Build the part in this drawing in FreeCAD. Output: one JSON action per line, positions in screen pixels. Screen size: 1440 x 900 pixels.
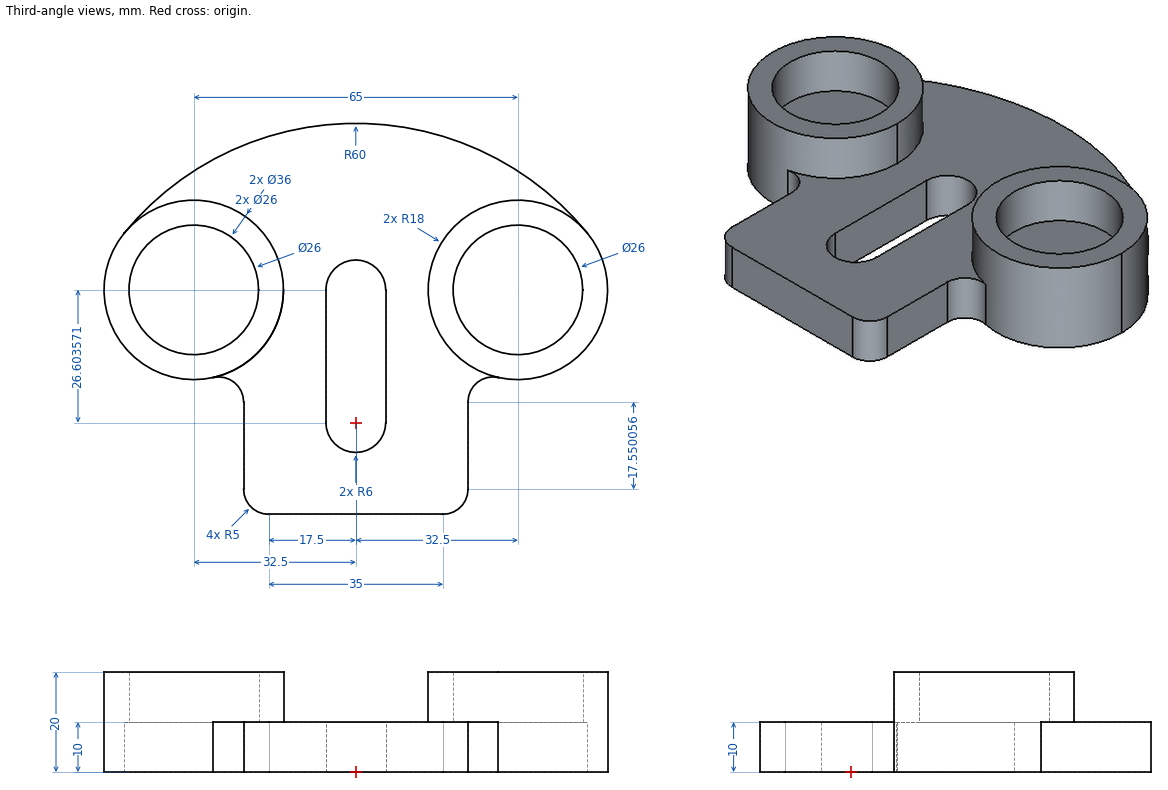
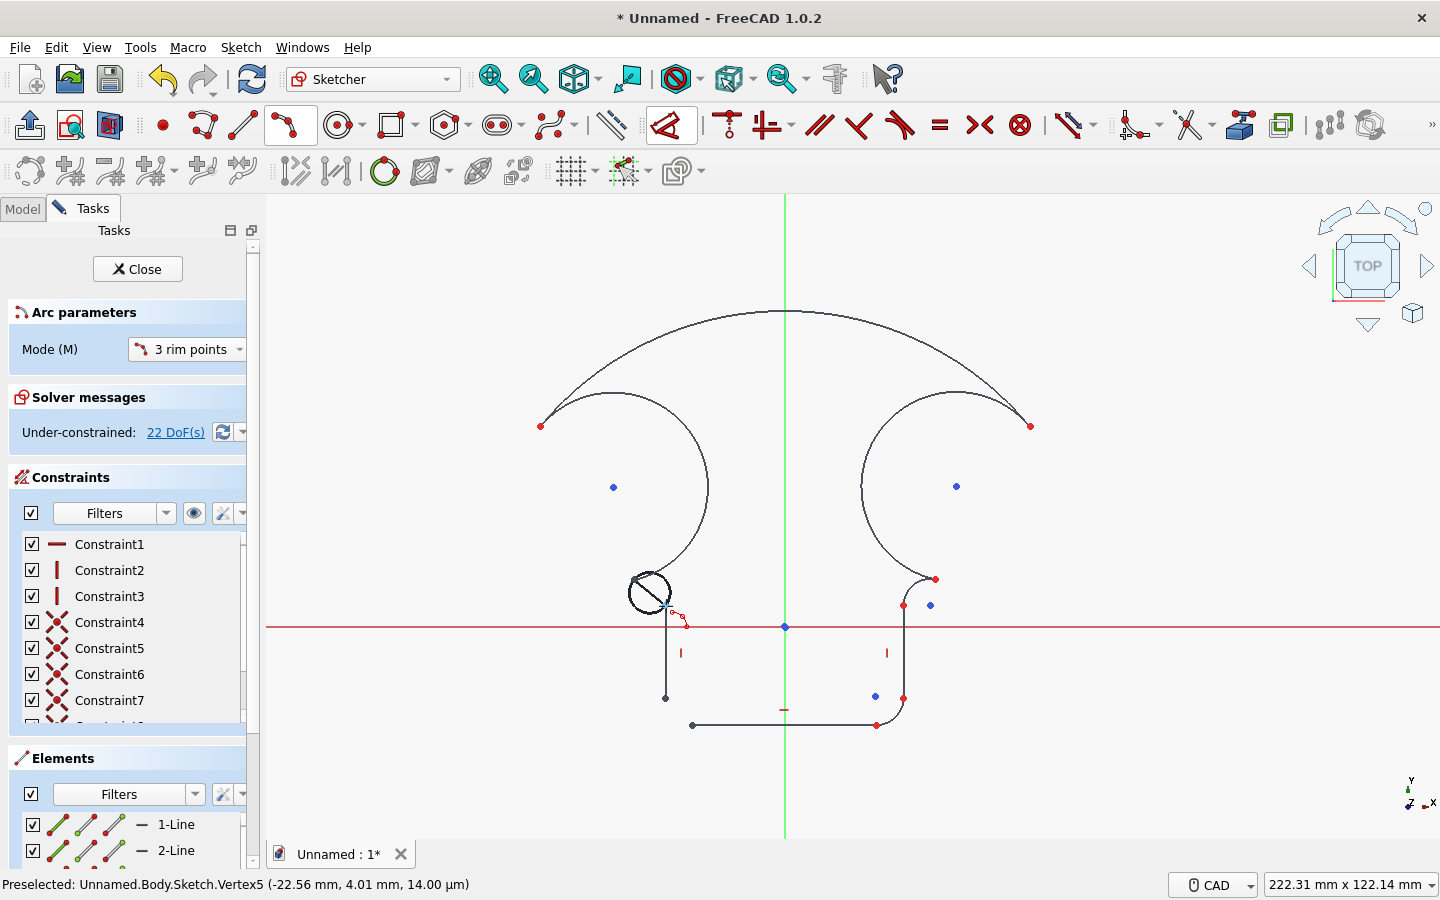
{"action": "scroll", "coordinate": [656, 584], "scroll_direction": "up", "scroll_amount": 3}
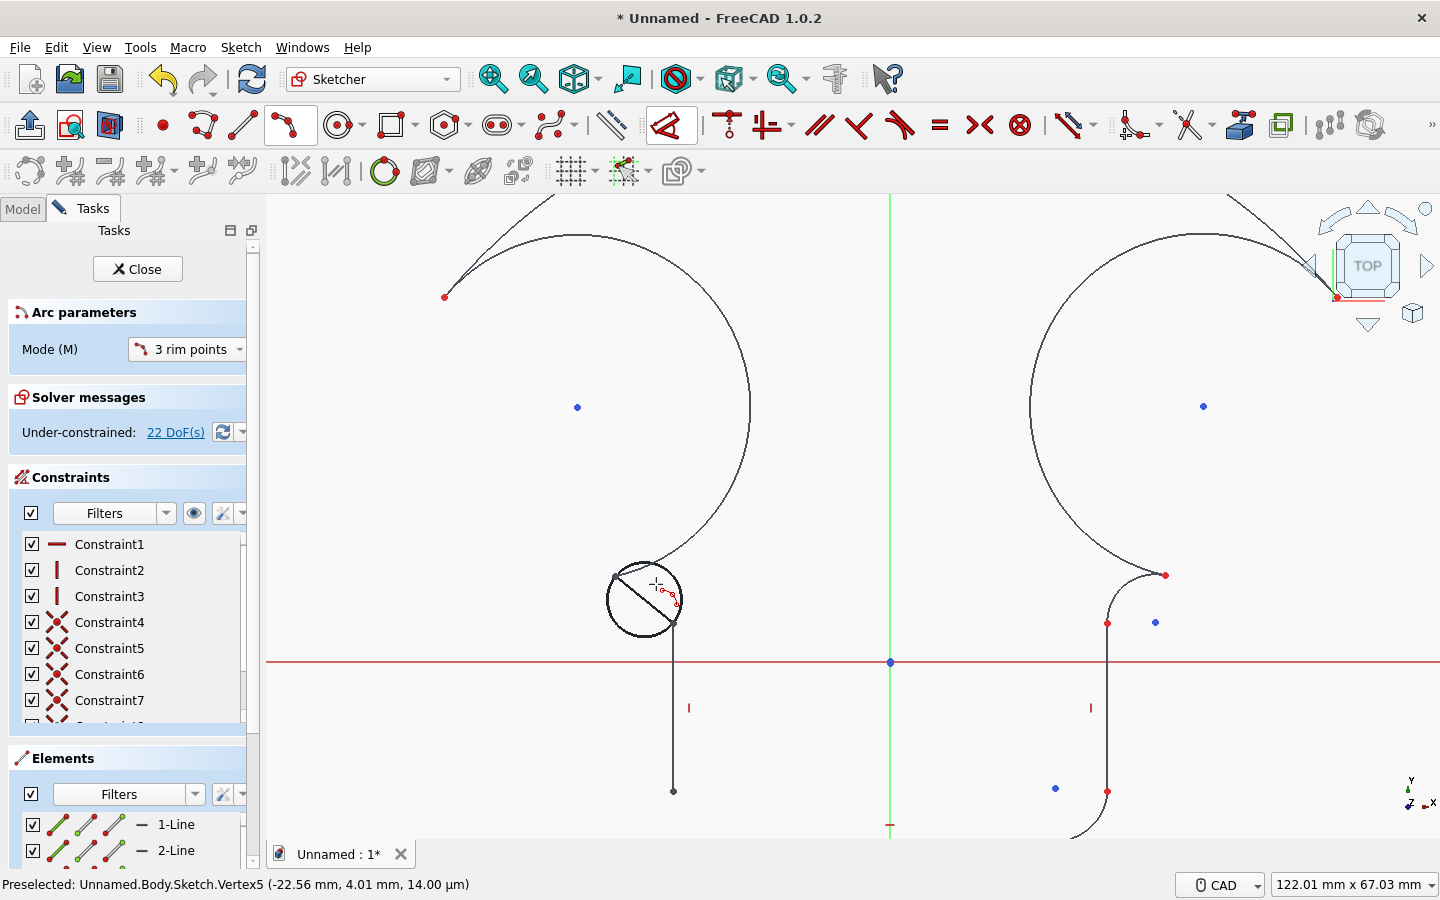
{"action": "left_click", "coordinate": [656, 584]}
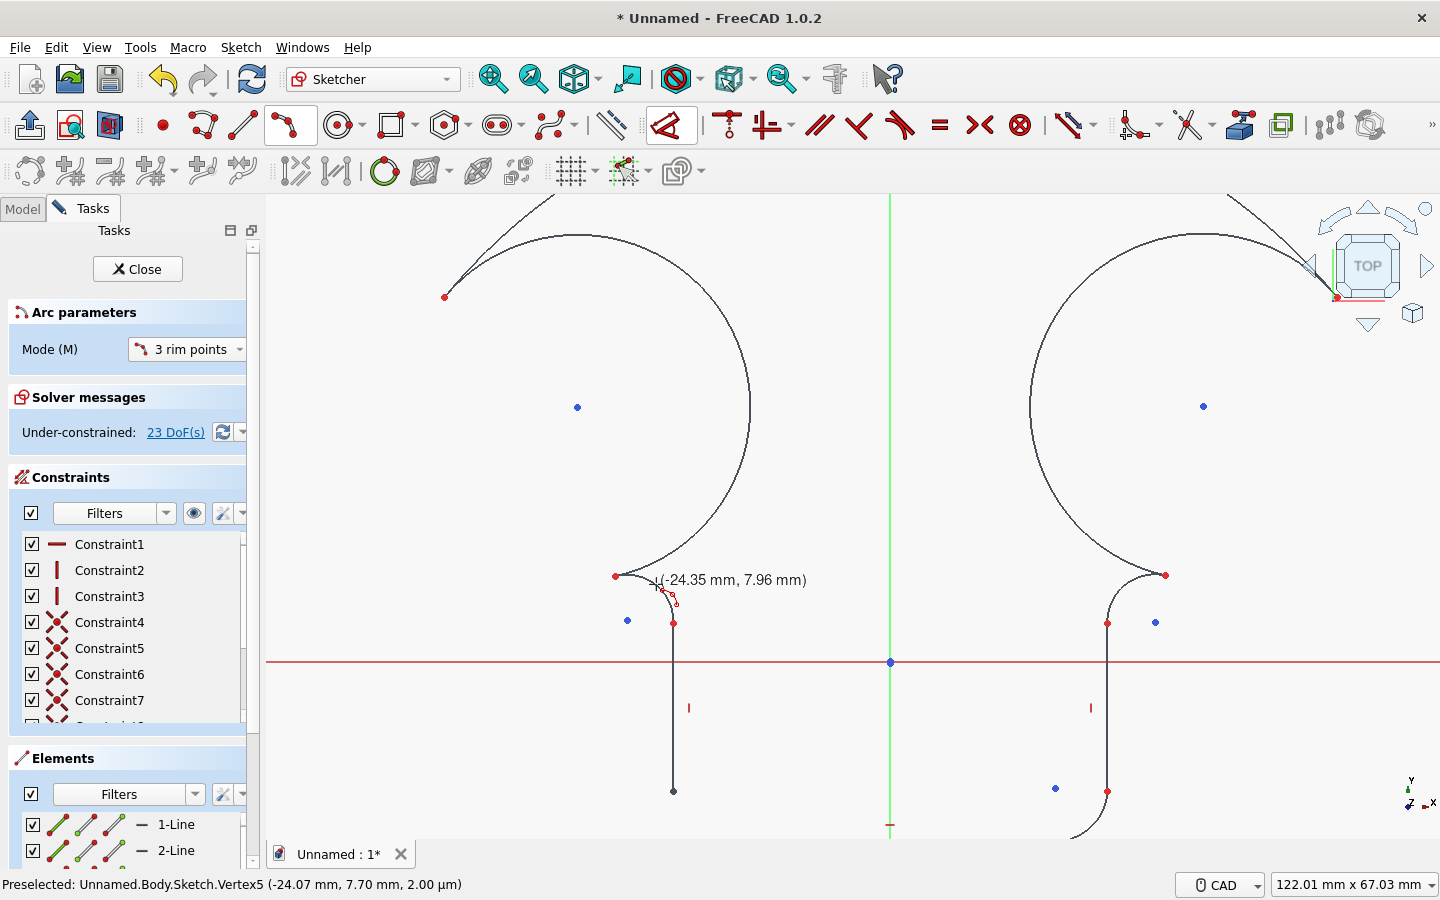
{"action": "left_click", "coordinate": [673, 792]}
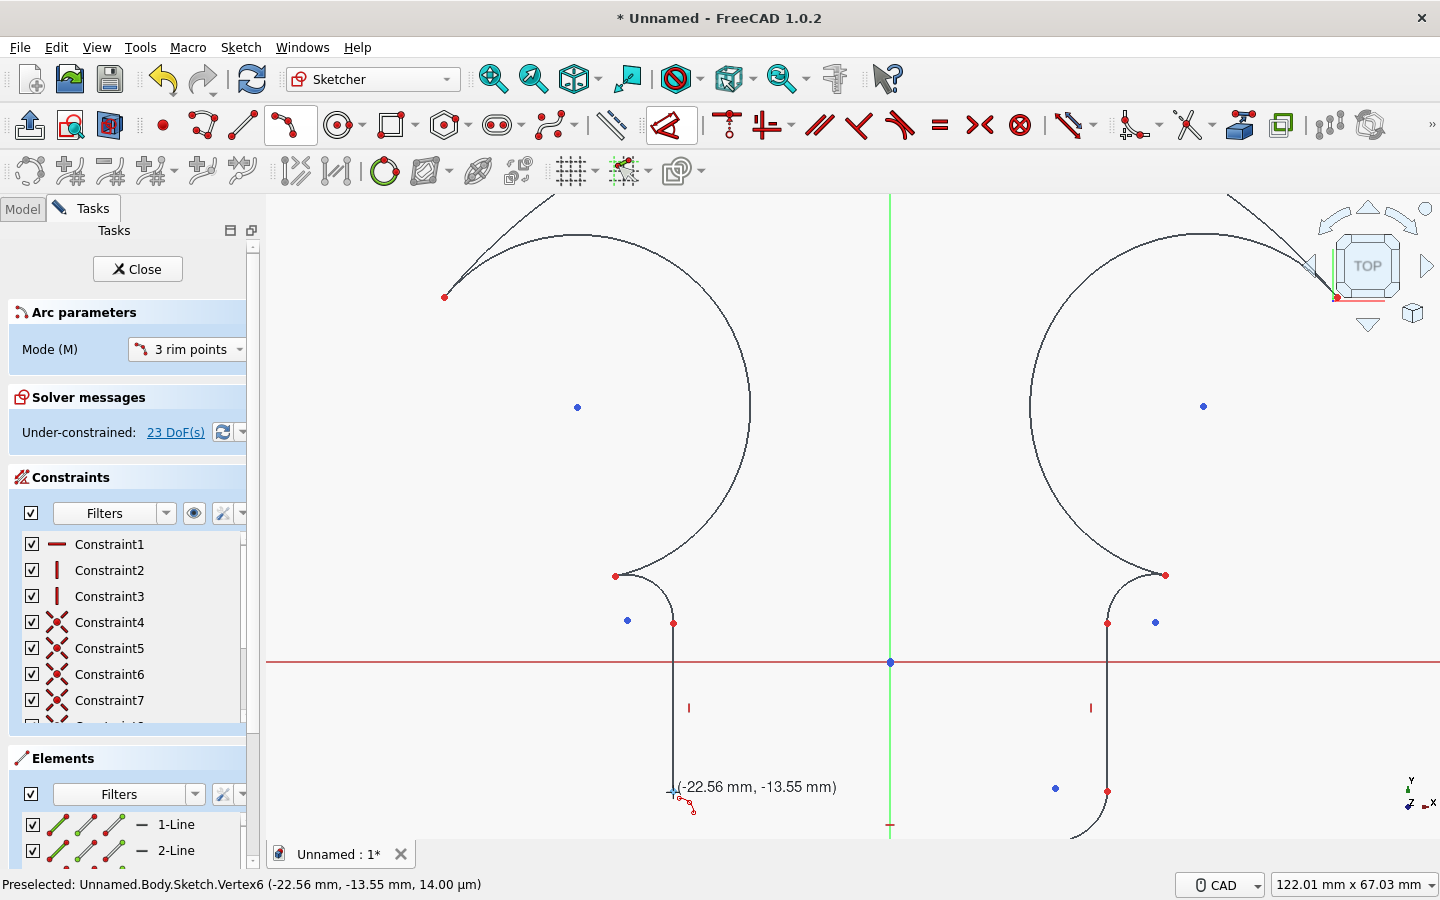
{"action": "scroll", "coordinate": [656, 583], "scroll_direction": "down", "scroll_amount": 3}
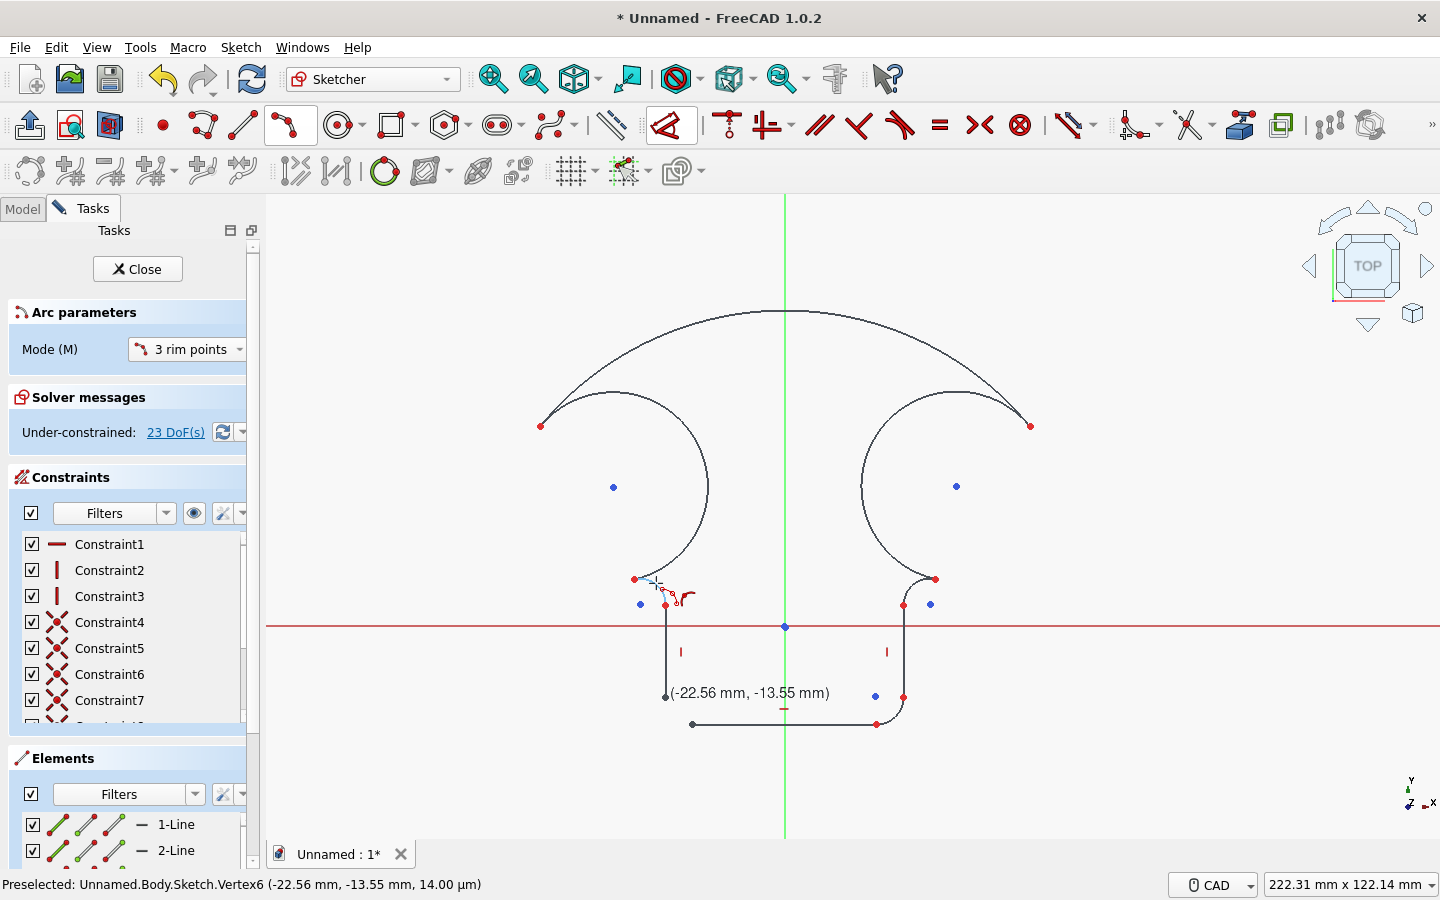
{"action": "left_click", "coordinate": [692, 725]}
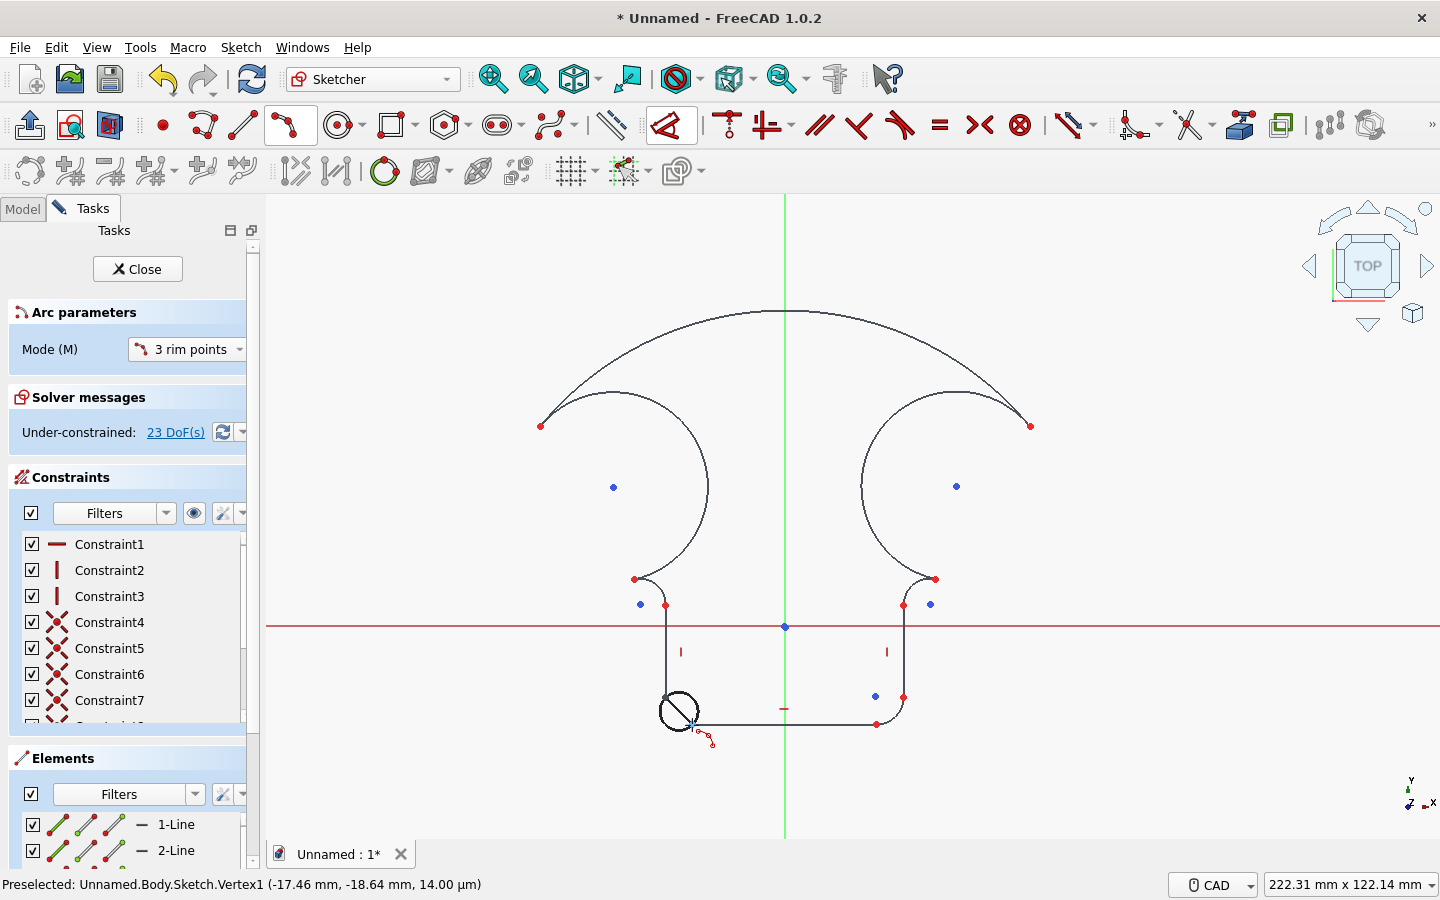
{"action": "scroll", "coordinate": [674, 716], "scroll_direction": "up", "scroll_amount": 4}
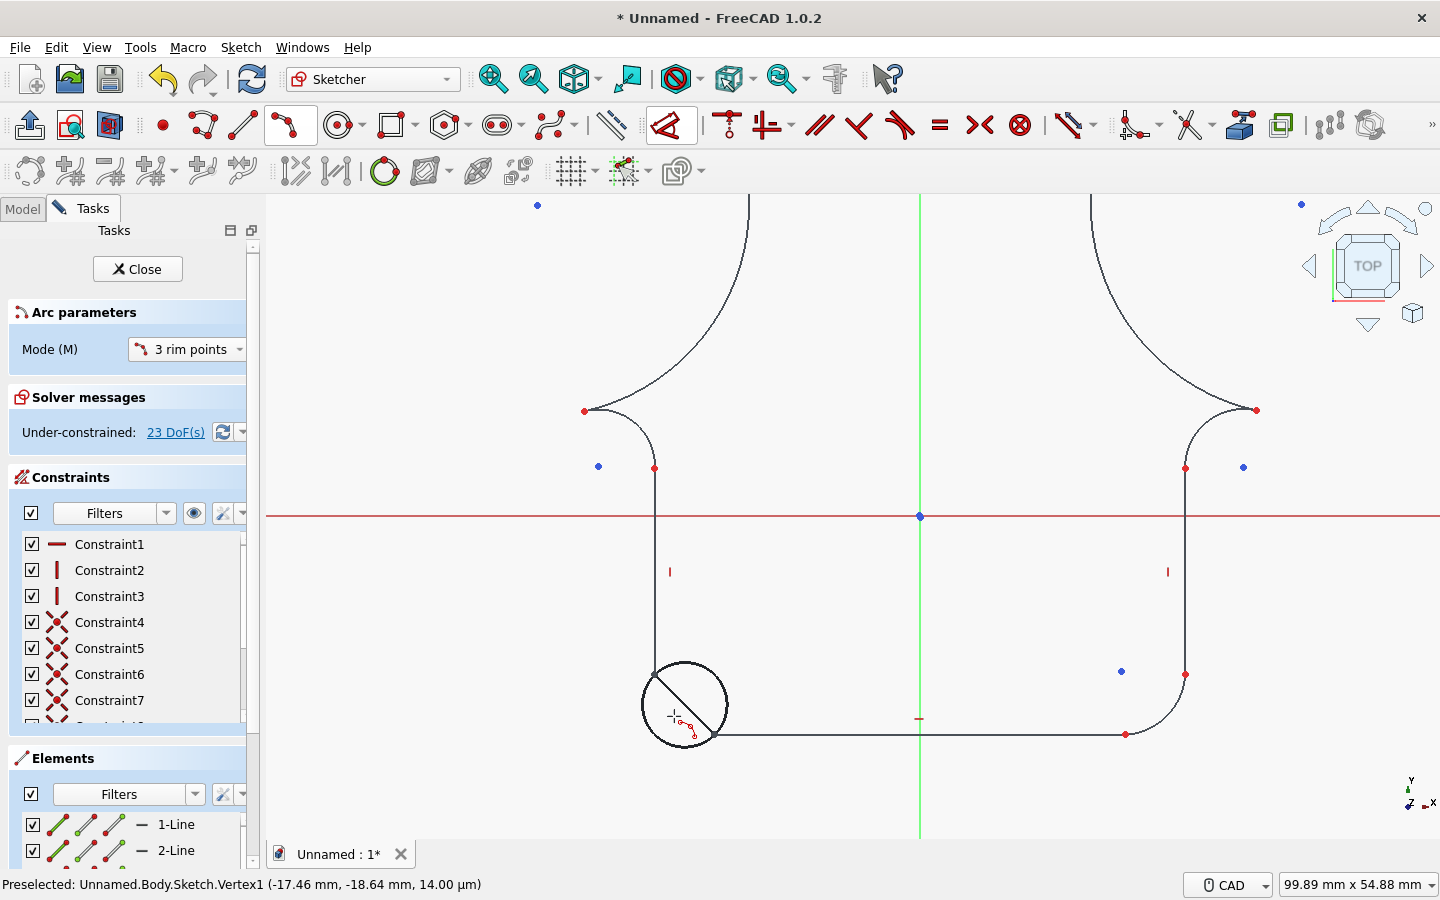
{"action": "left_click", "coordinate": [673, 715]}